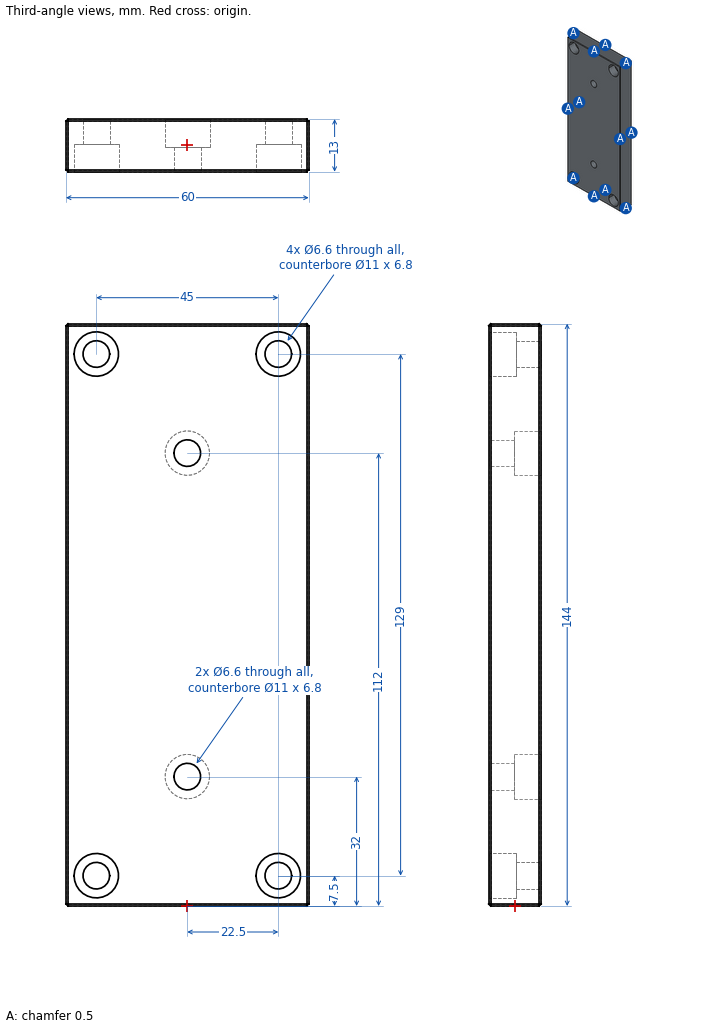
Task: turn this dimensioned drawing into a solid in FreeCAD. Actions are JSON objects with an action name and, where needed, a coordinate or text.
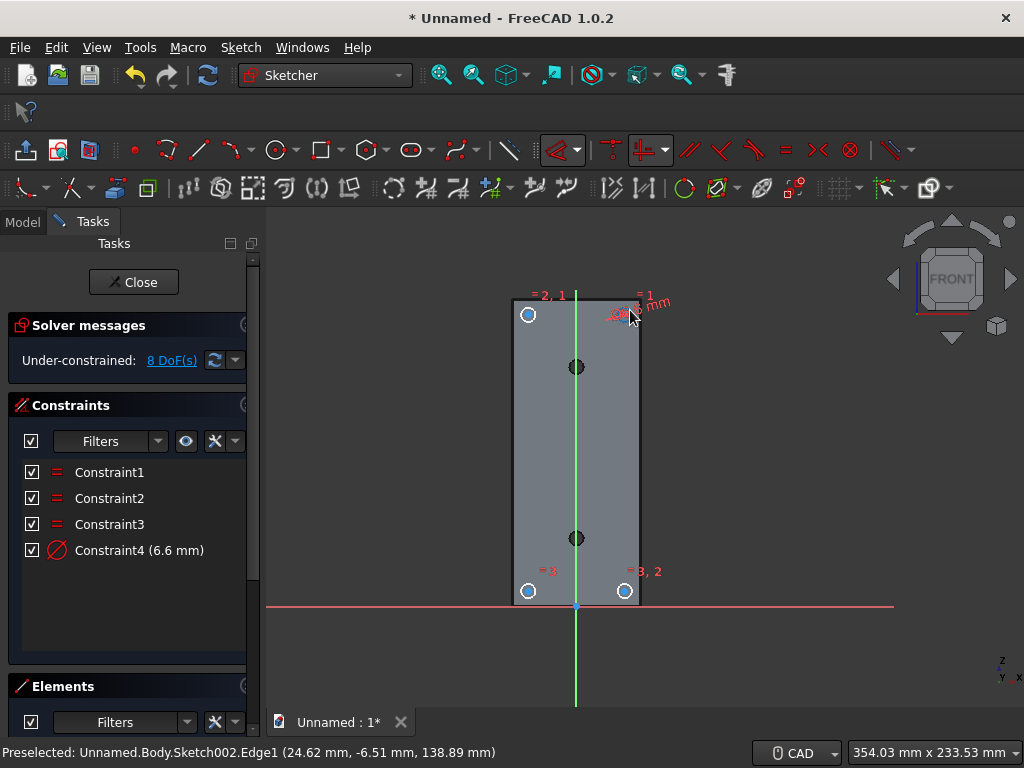
{"action": "scroll", "coordinate": [625, 591], "scroll_direction": "up", "scroll_amount": 5}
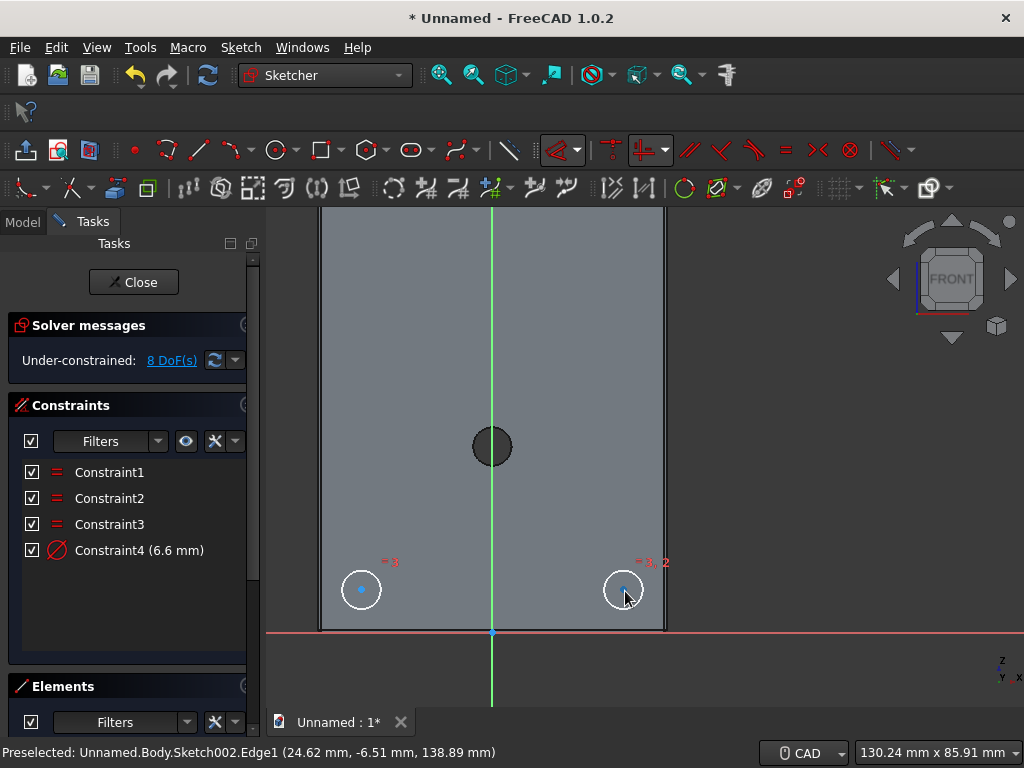
{"action": "left_click", "coordinate": [623, 590]}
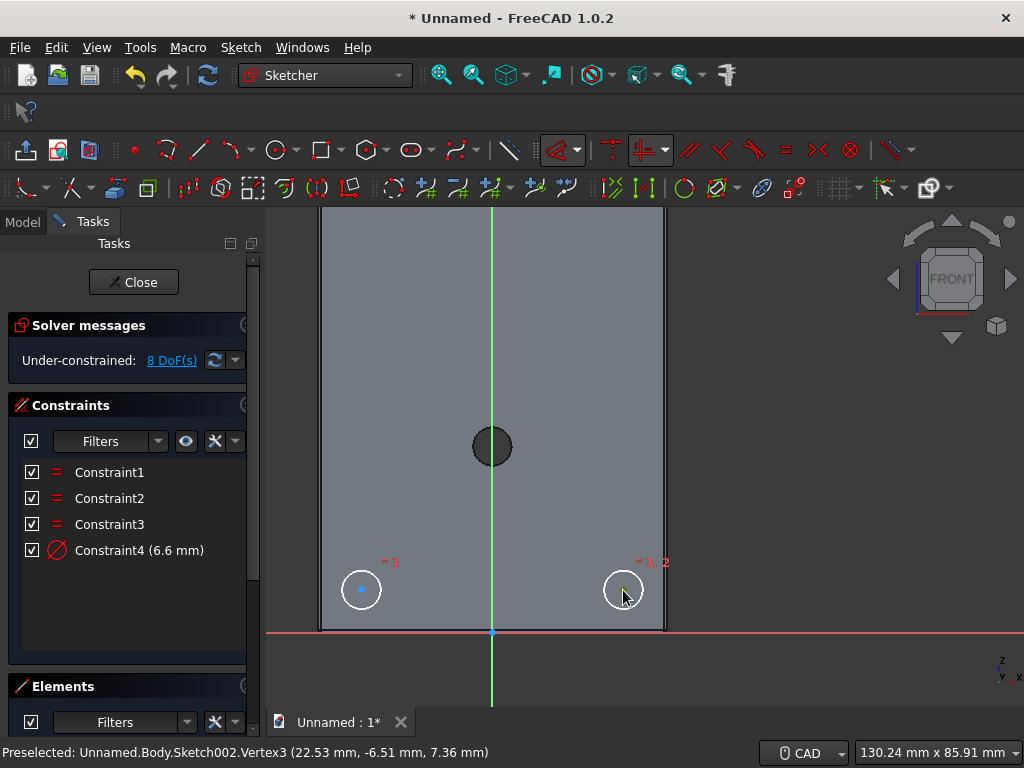
{"action": "key", "text": "i"}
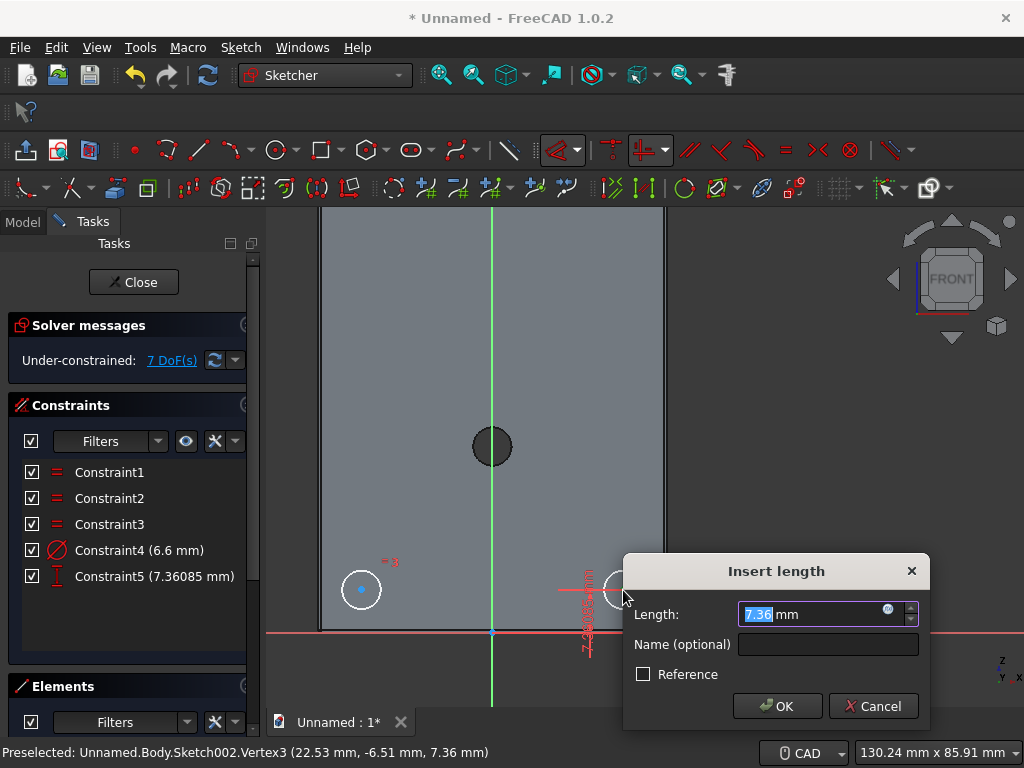
{"action": "type", "text": "7.5"}
{"action": "key", "text": "Return"}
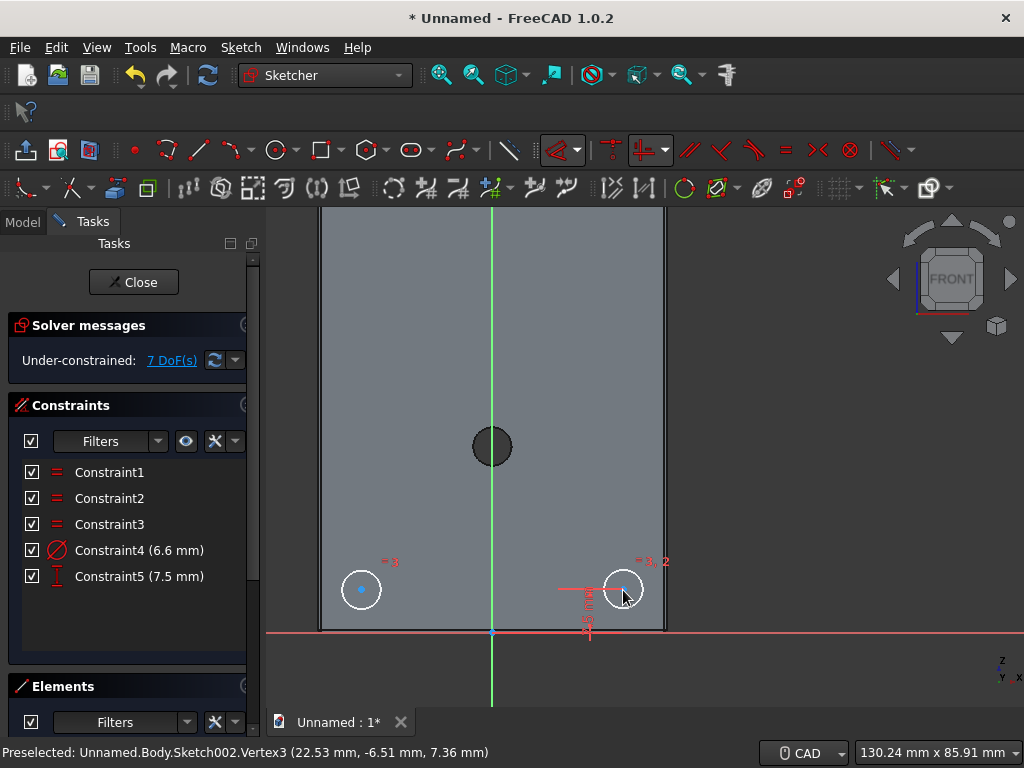
{"action": "left_click", "coordinate": [361, 590]}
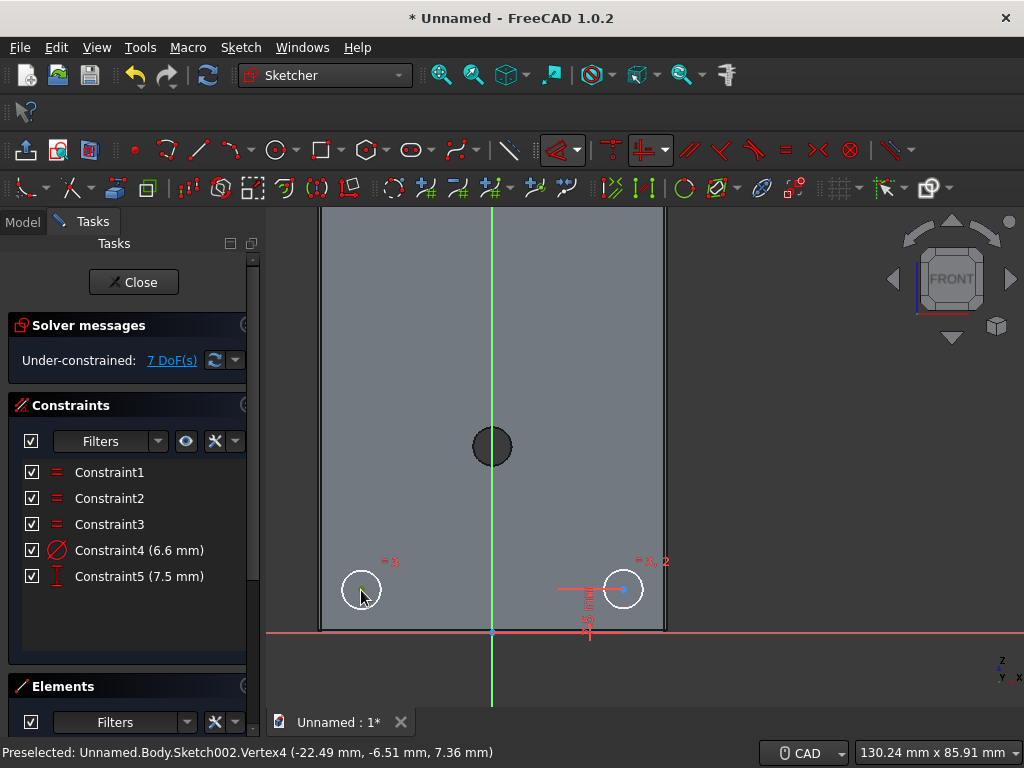
{"action": "key", "text": "i"}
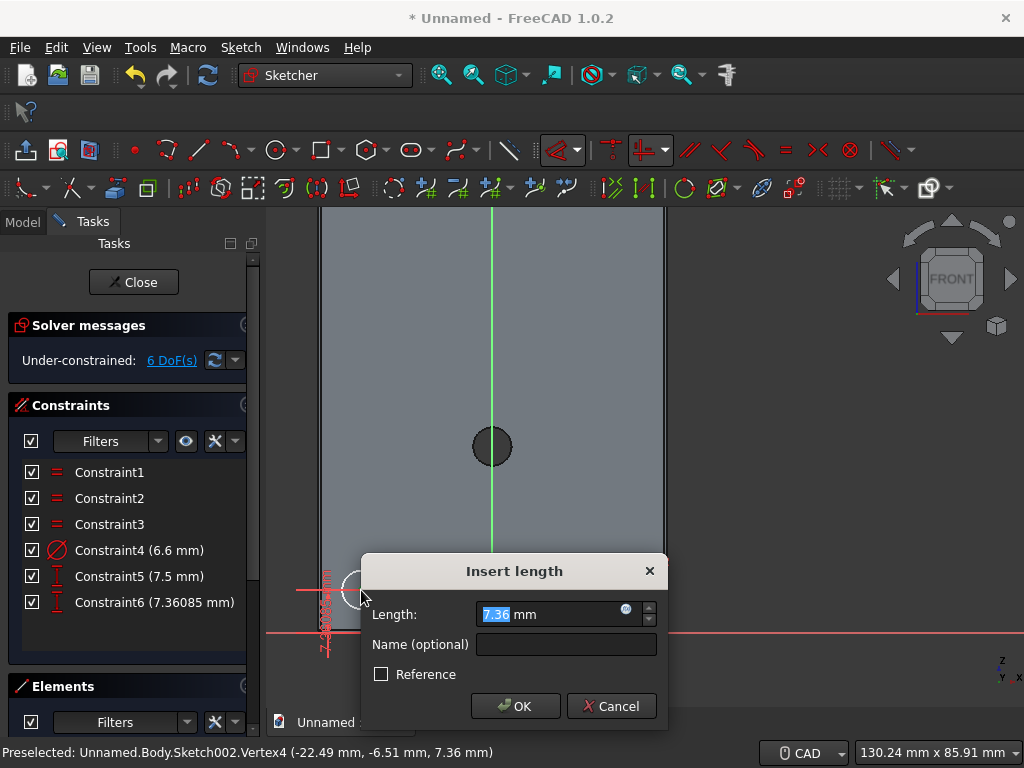
{"action": "type", "text": "7.5"}
{"action": "key", "text": "Return"}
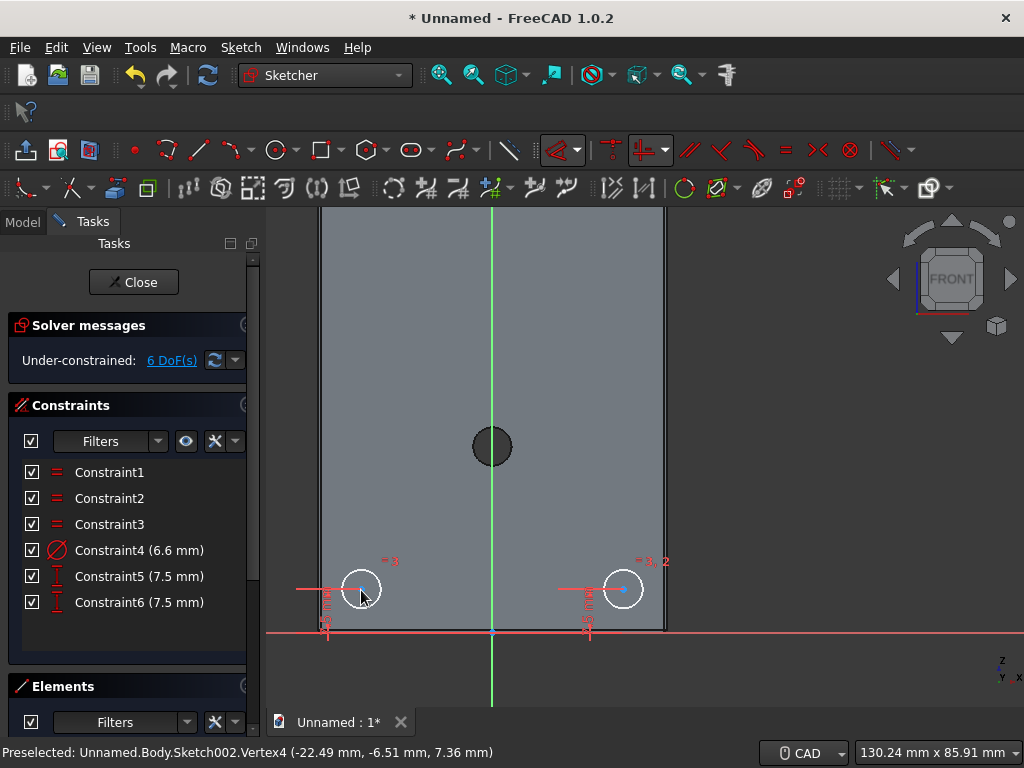
{"action": "scroll", "coordinate": [625, 591], "scroll_direction": "down", "scroll_amount": 5}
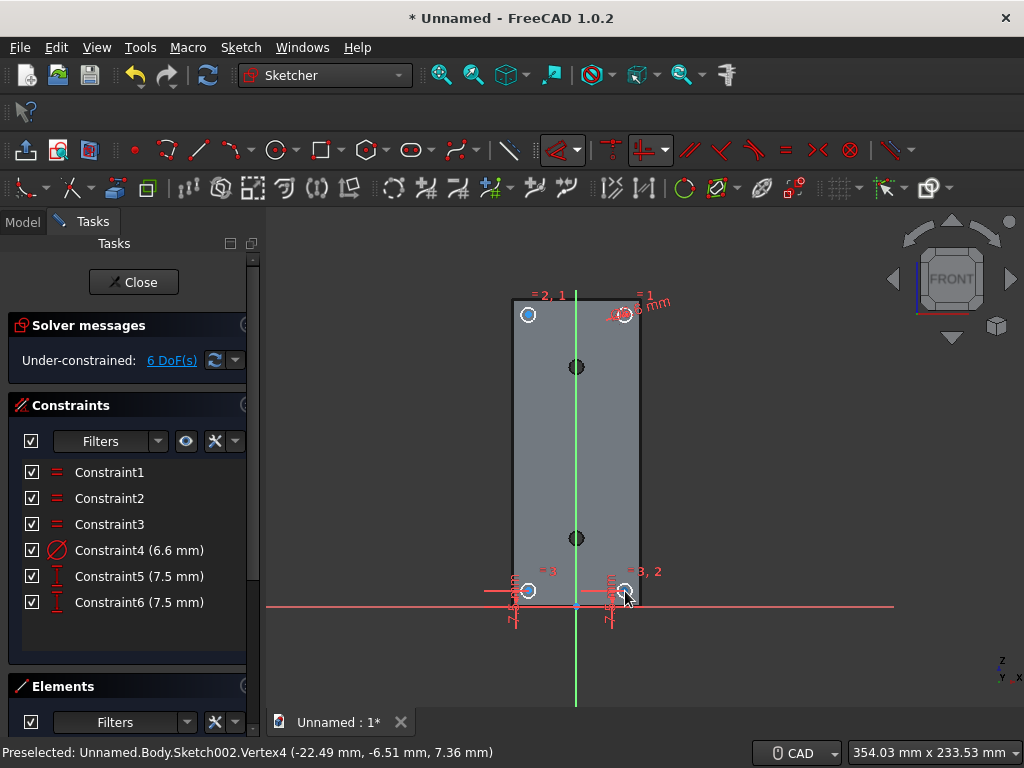
{"action": "left_click", "coordinate": [625, 315]}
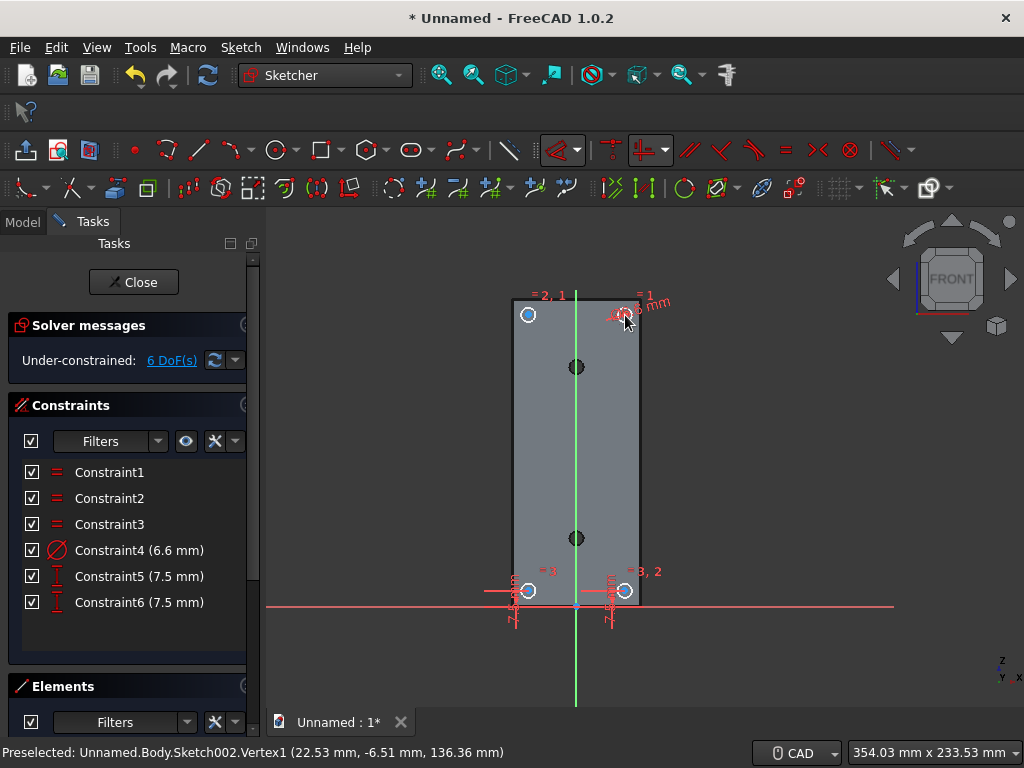
{"action": "left_click", "coordinate": [528, 315]}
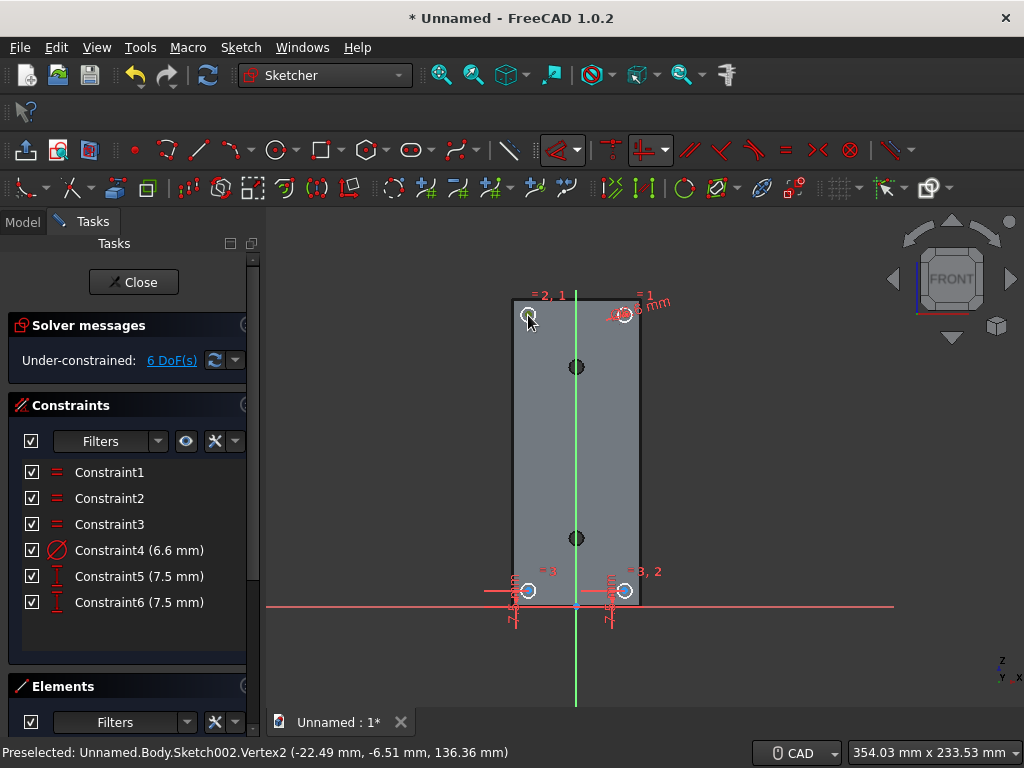
{"action": "left_click", "coordinate": [580, 150]}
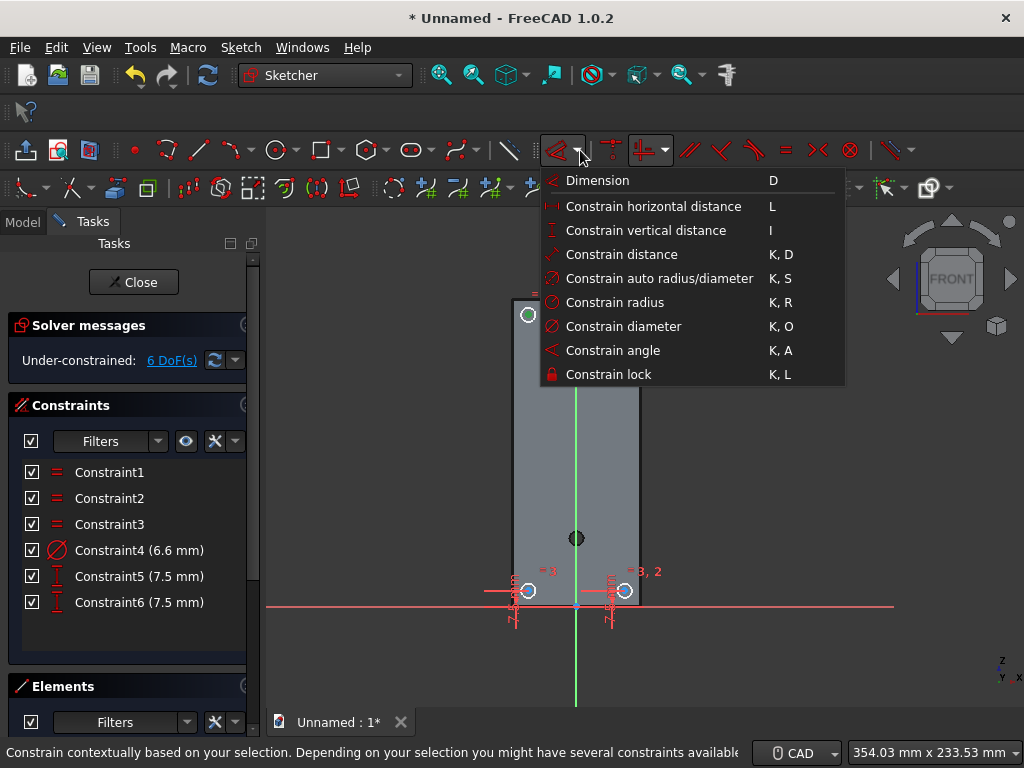
{"action": "left_click", "coordinate": [693, 206]}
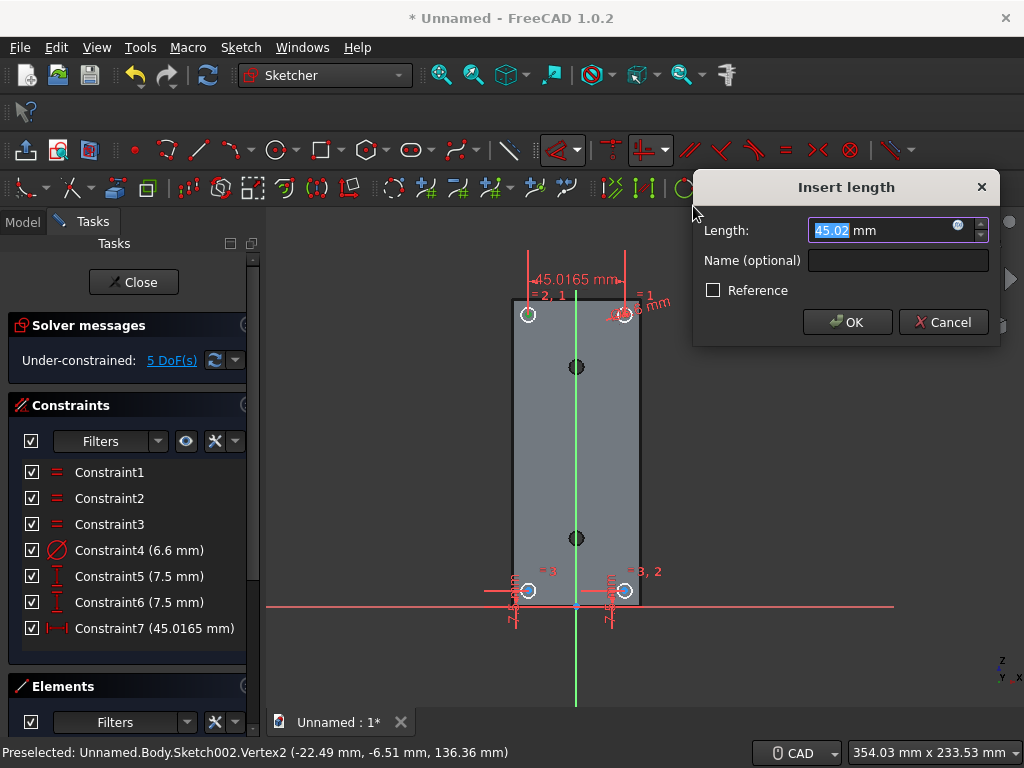
{"action": "type", "text": "45"}
{"action": "key", "text": "Return"}